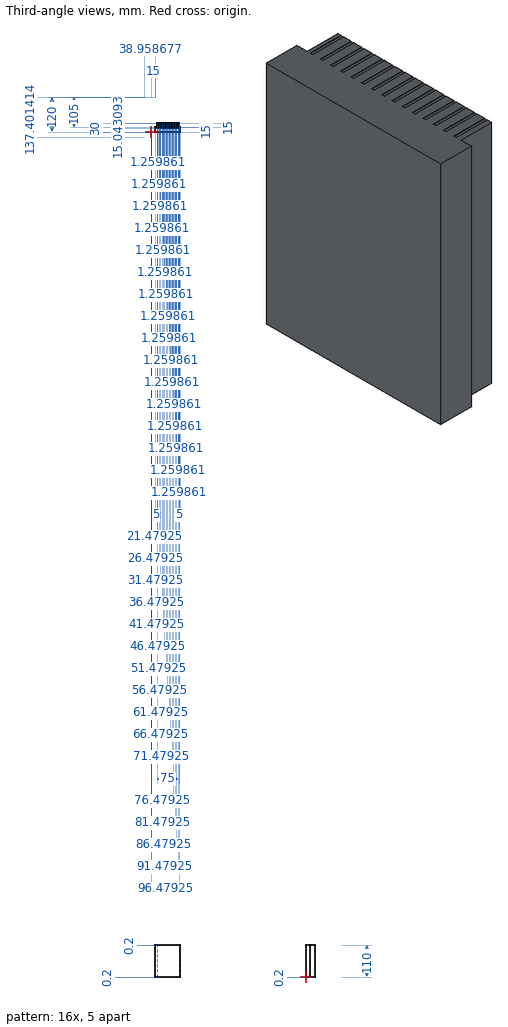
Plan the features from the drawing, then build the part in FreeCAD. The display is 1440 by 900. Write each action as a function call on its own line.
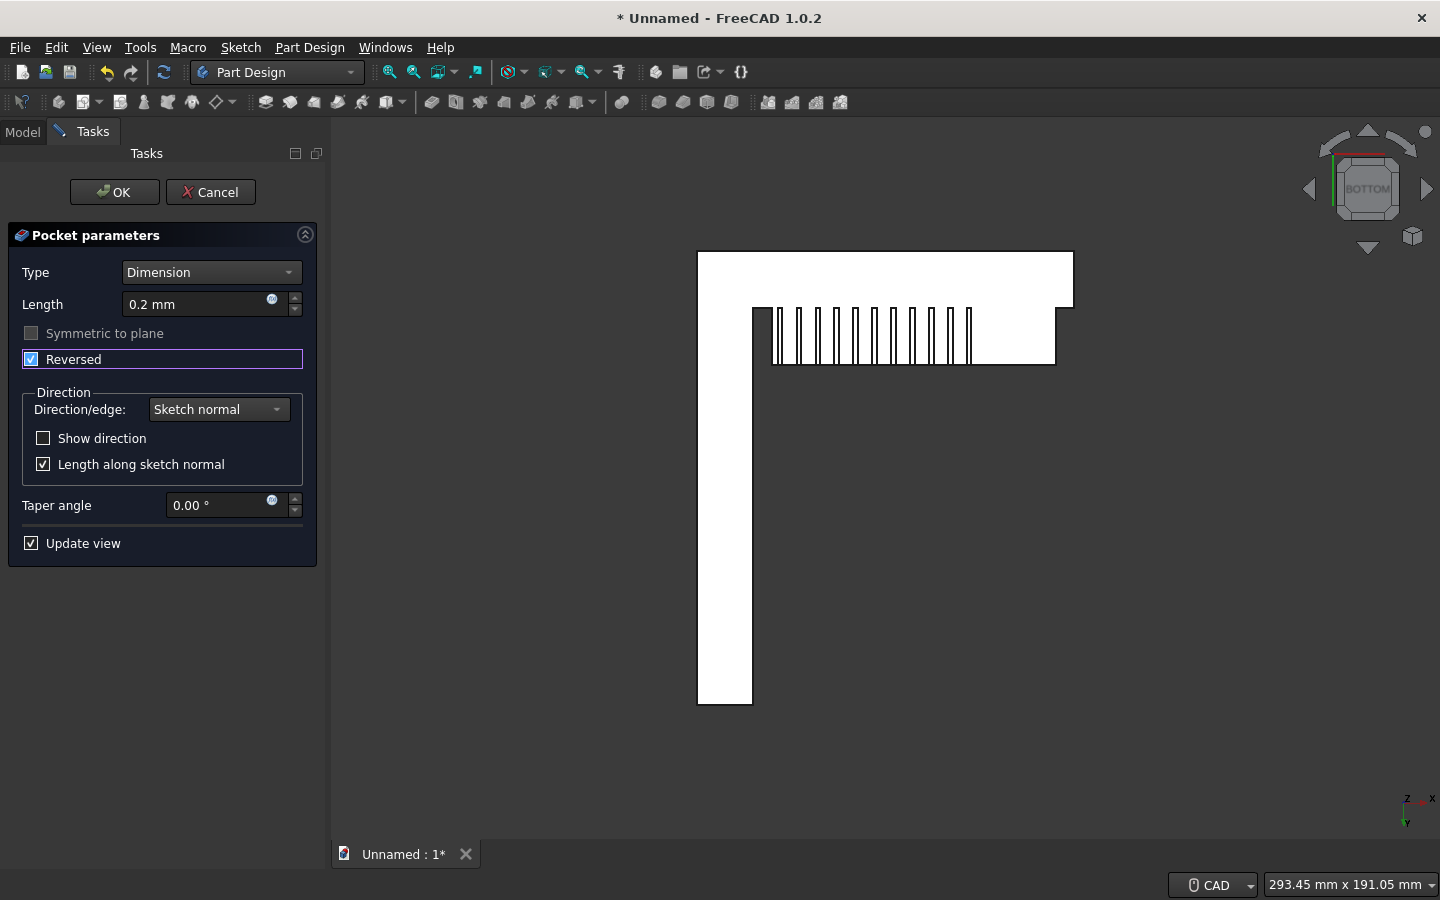
click(115, 192)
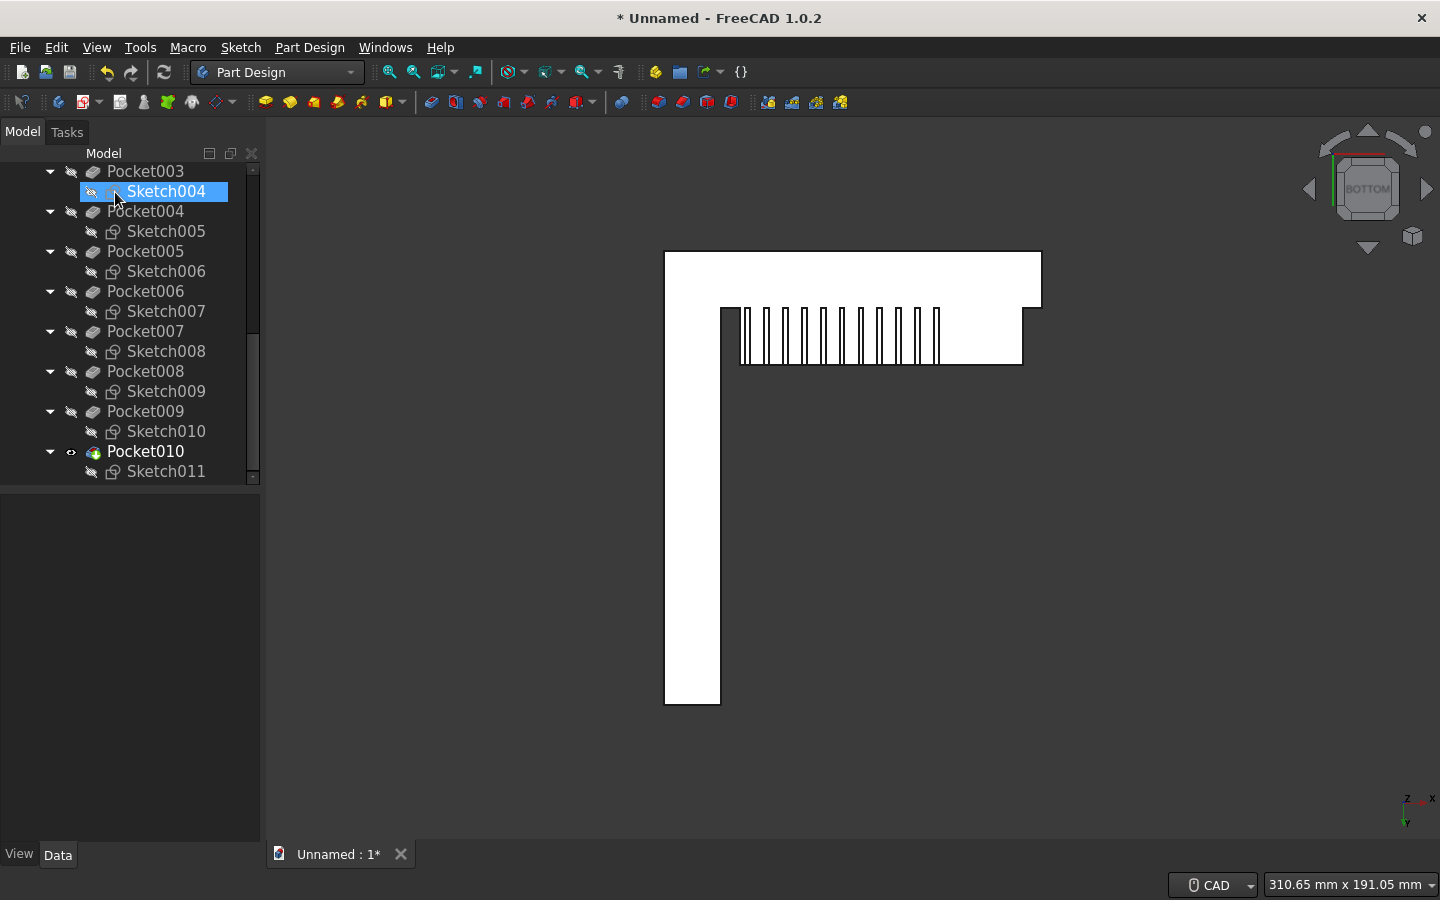
click(84, 102)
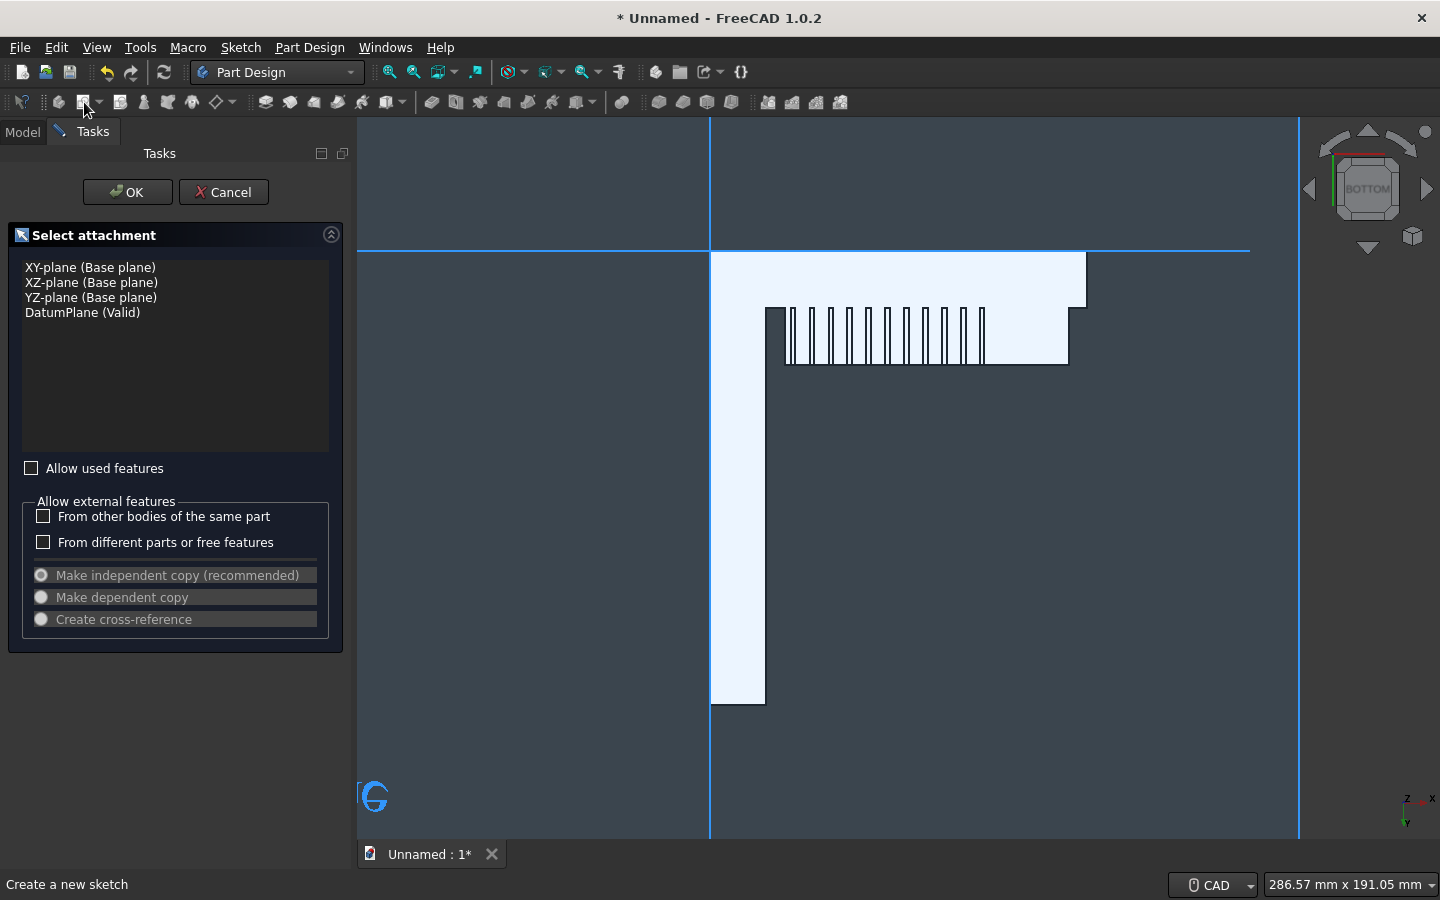
click(82, 268)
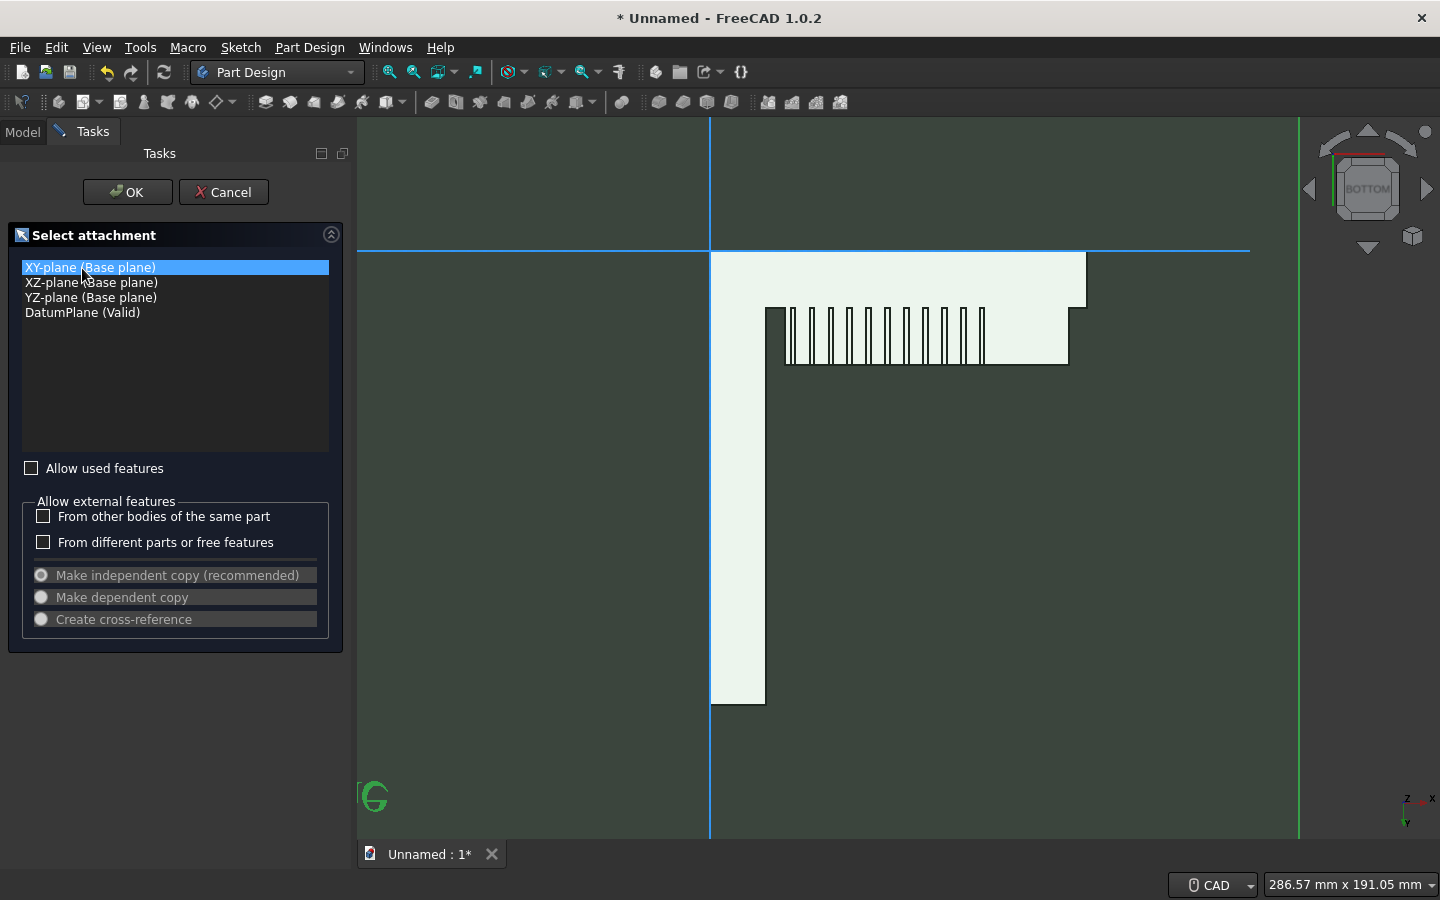
click(128, 192)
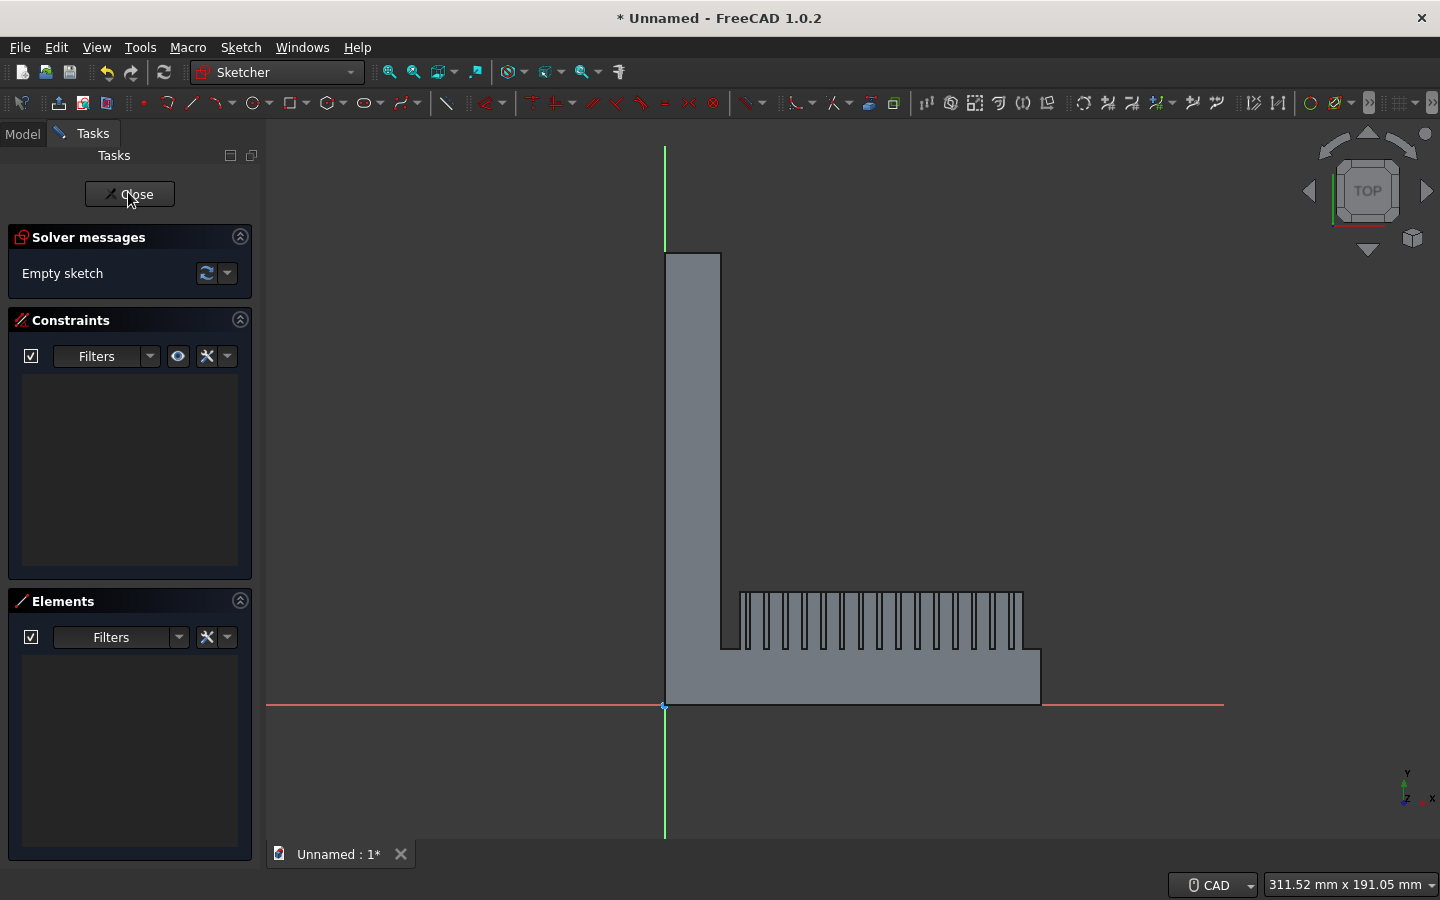
click(108, 104)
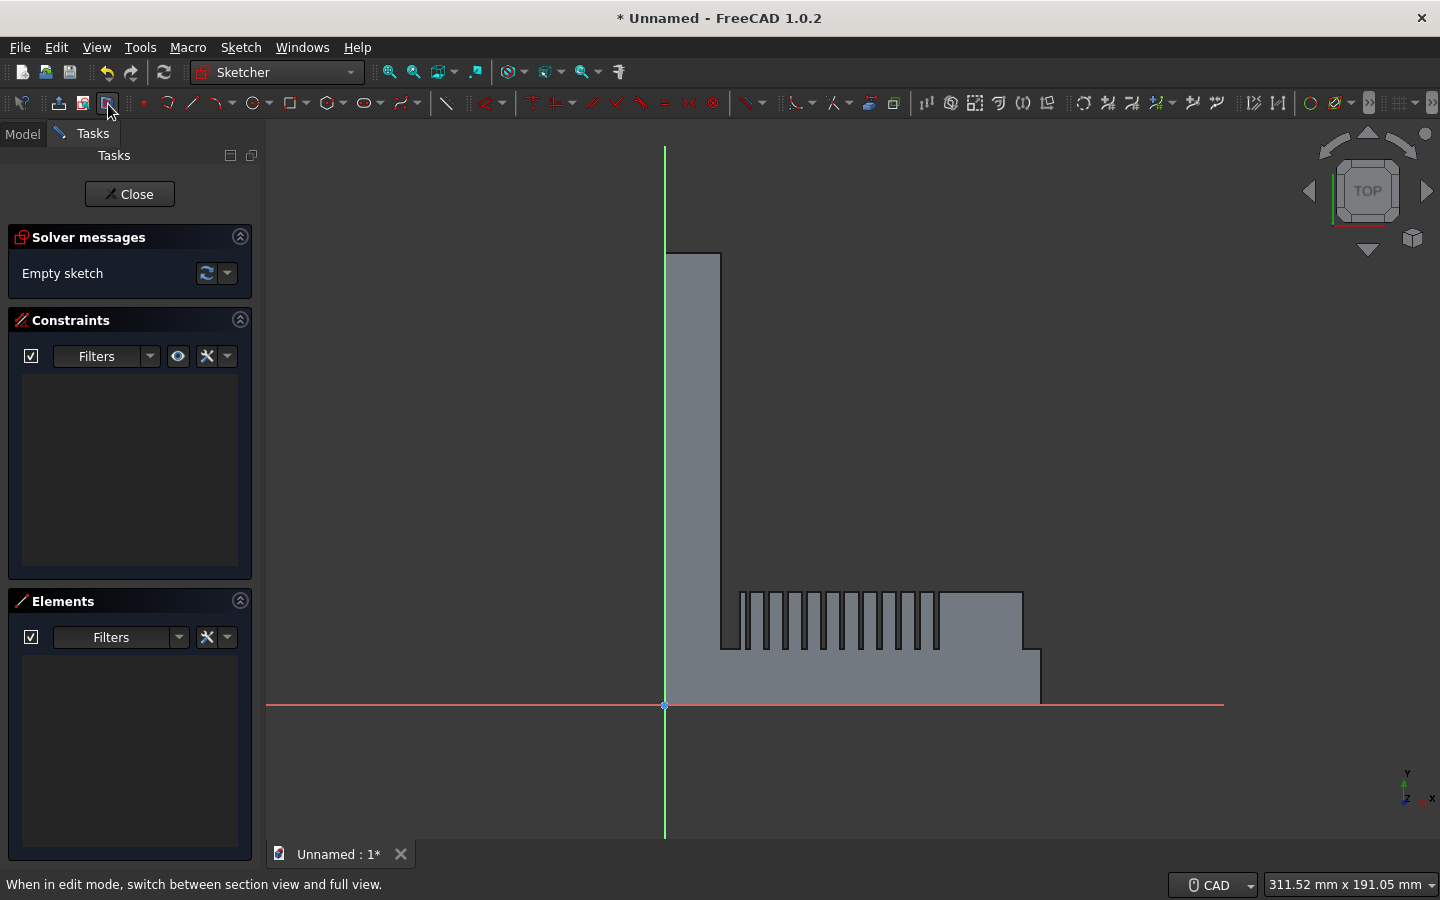
scroll(976, 638, up, 11)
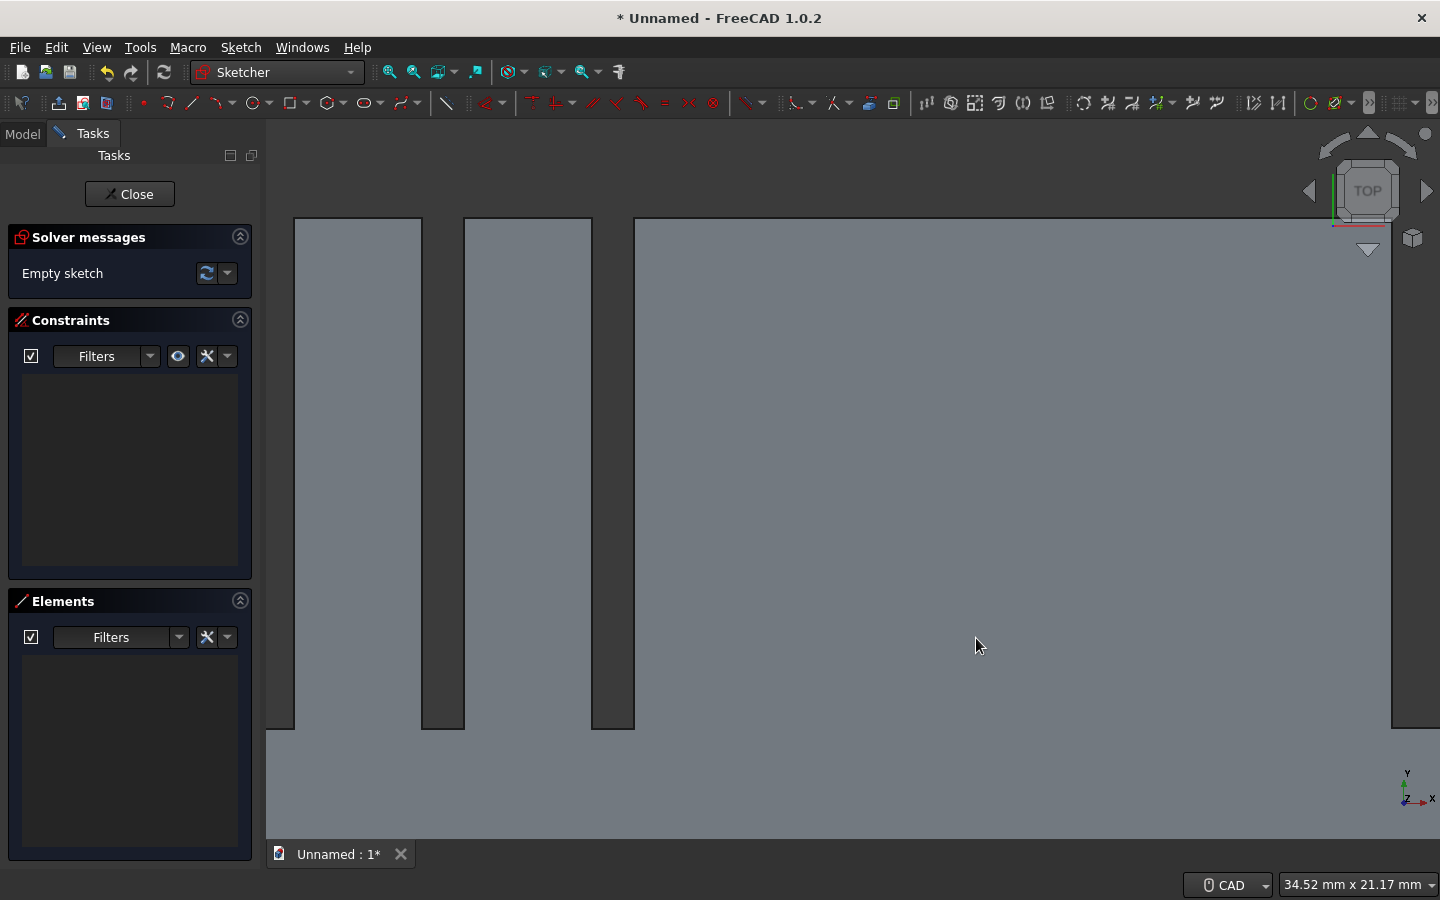
click(290, 104)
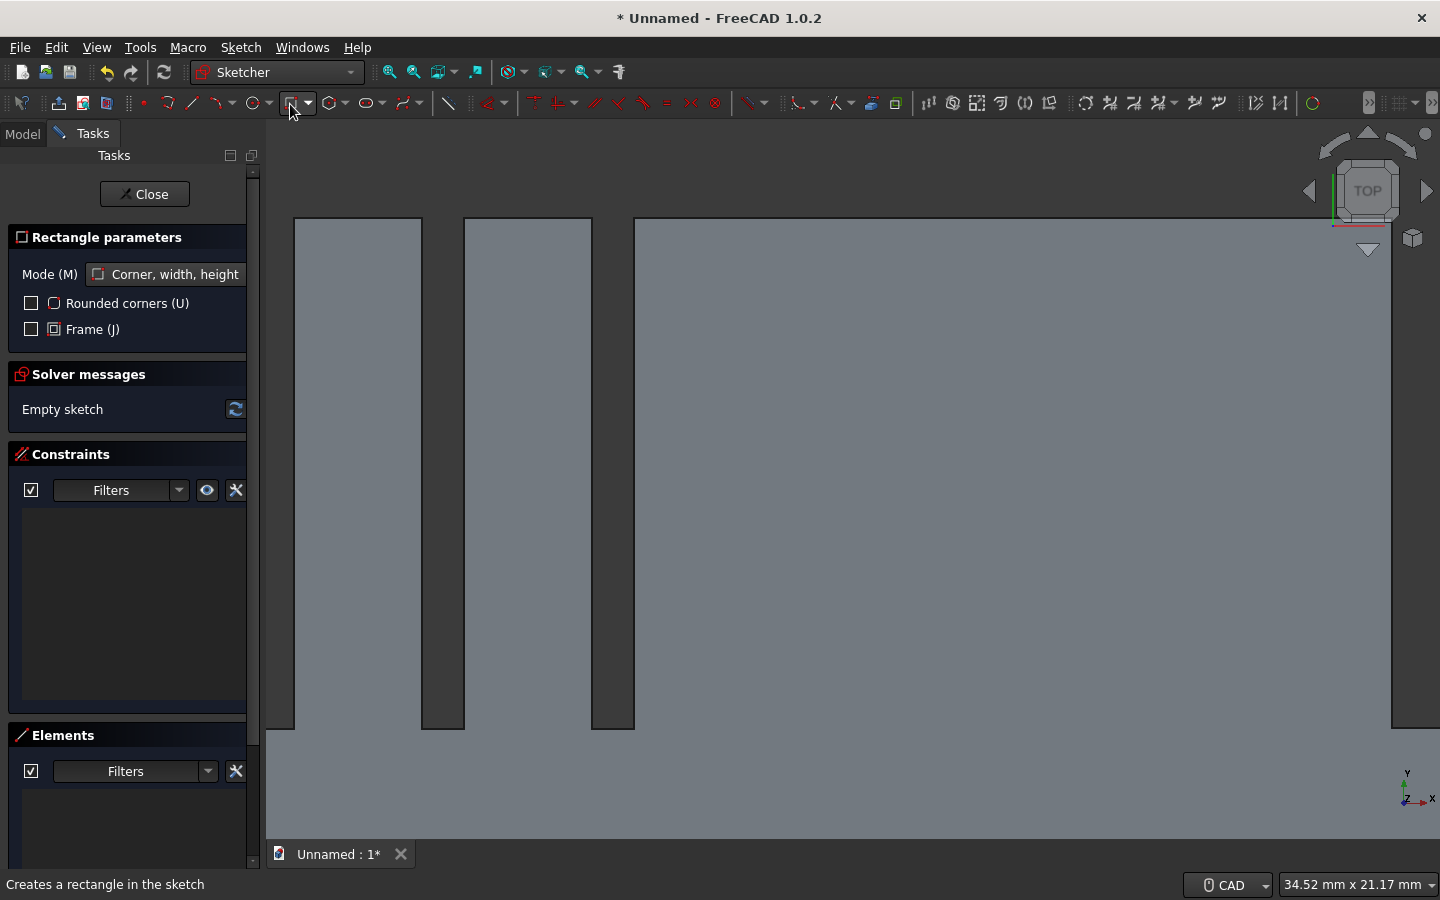
click(762, 218)
click(805, 729)
key(Escape)